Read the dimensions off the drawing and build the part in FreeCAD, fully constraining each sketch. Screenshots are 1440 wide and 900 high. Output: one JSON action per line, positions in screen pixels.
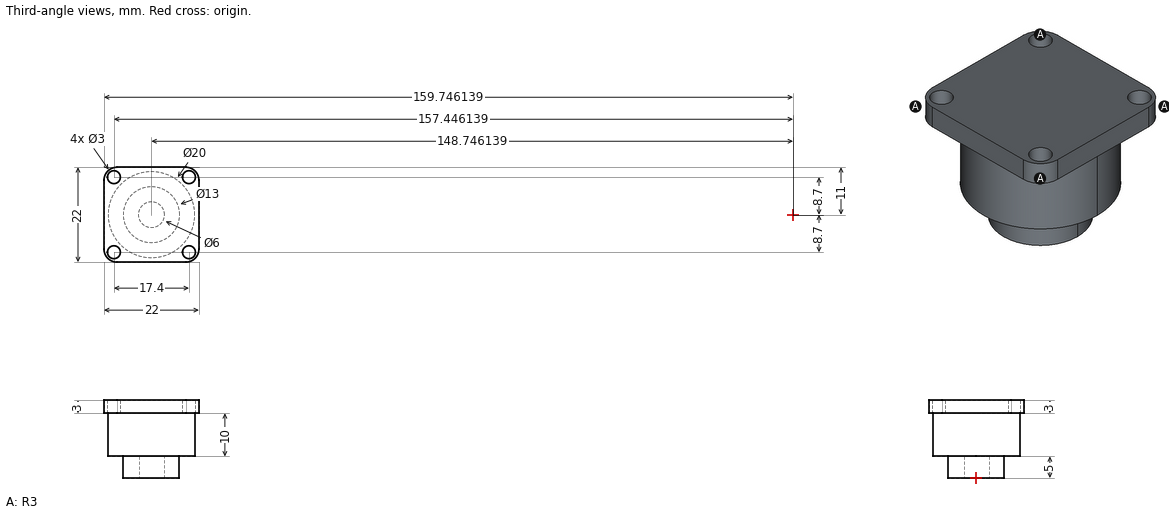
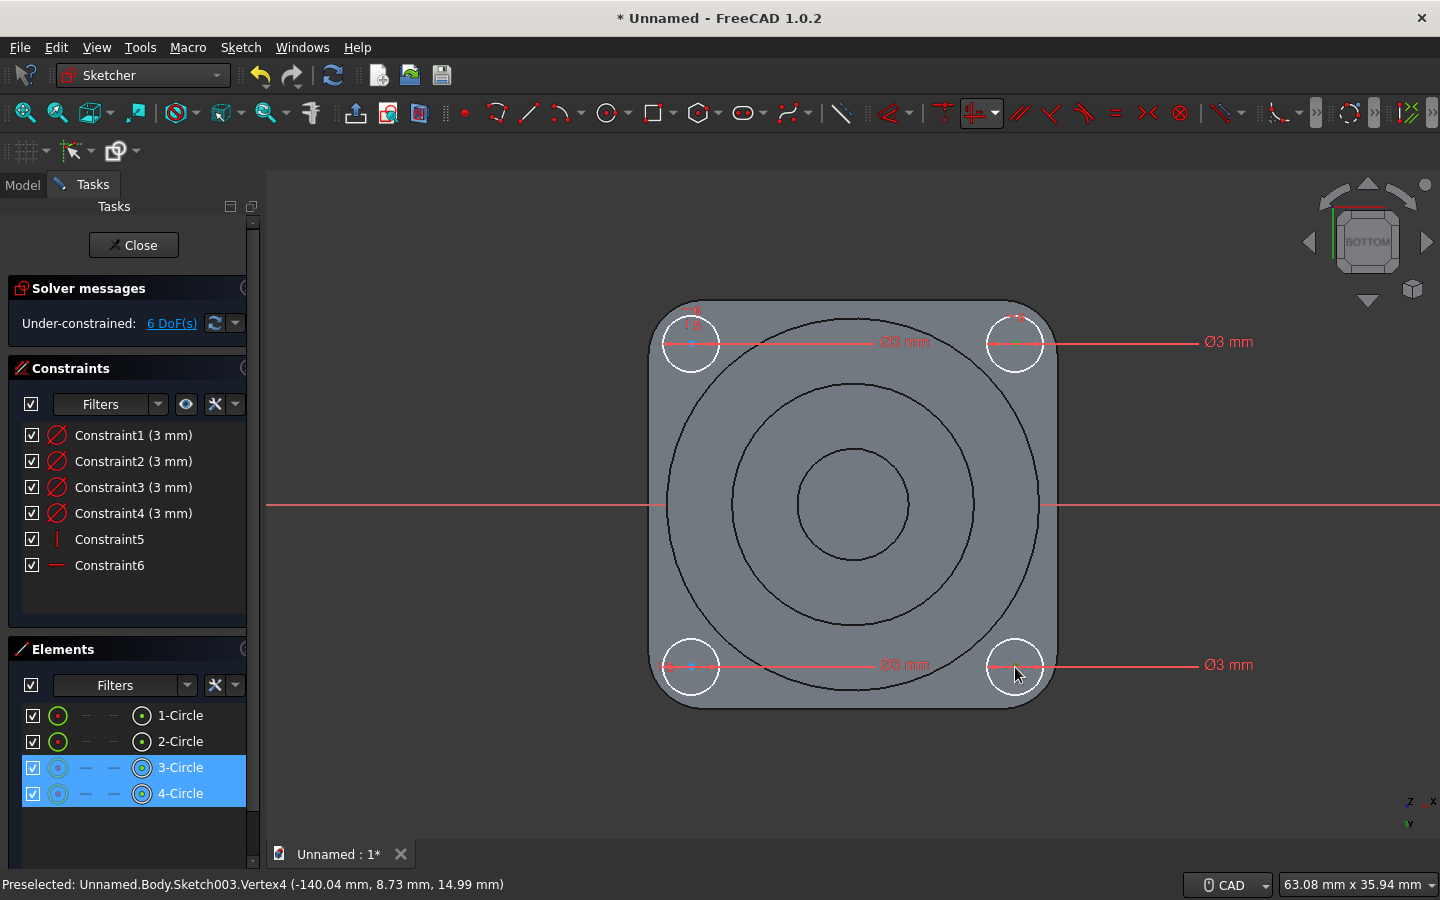
{"action": "left_click", "coordinate": [998, 114]}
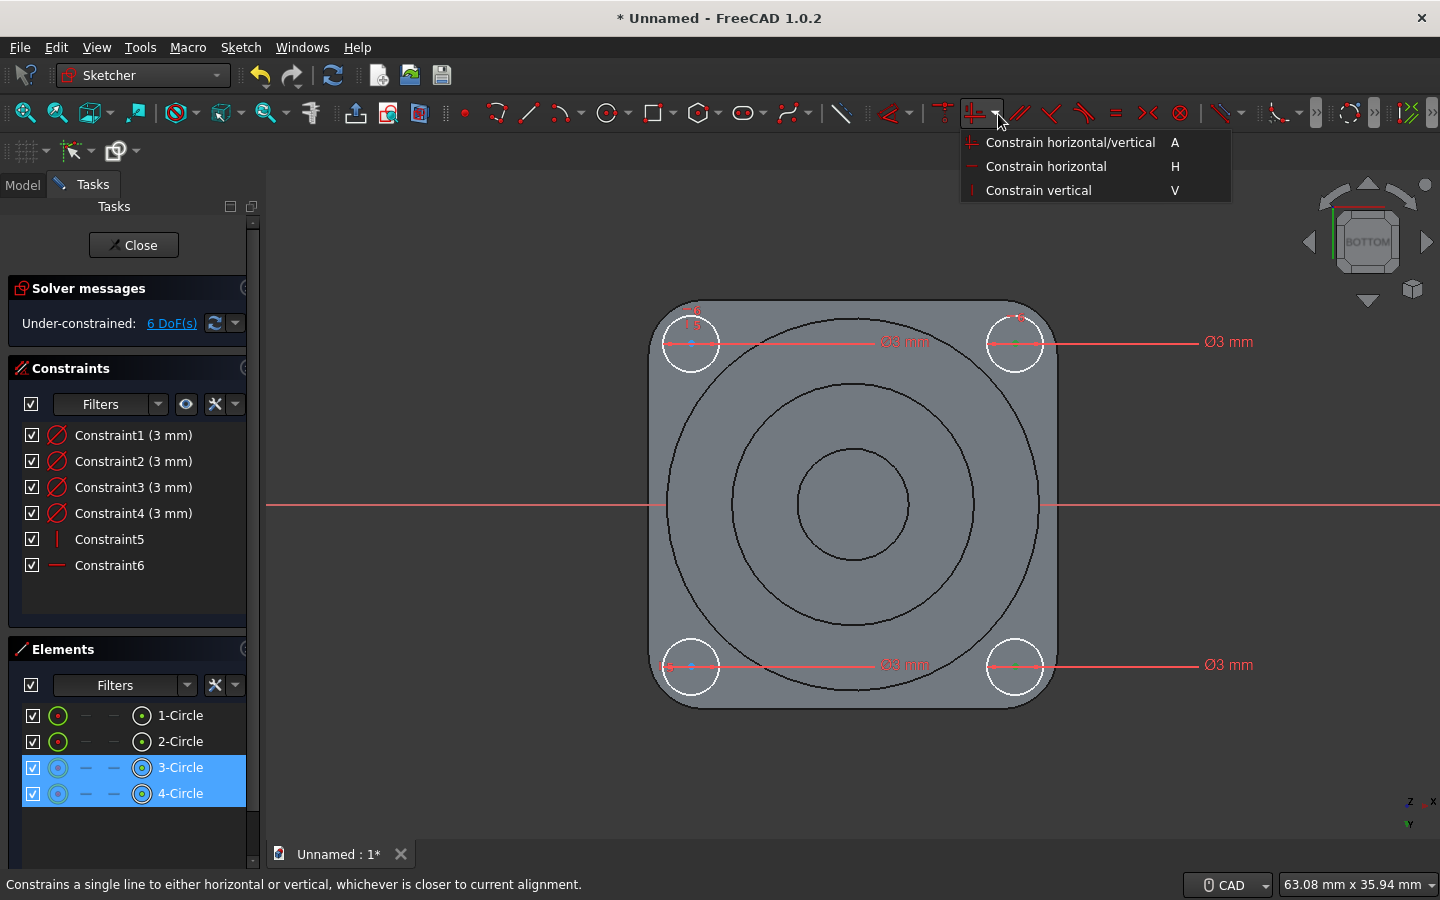
{"action": "left_click", "coordinate": [1096, 190]}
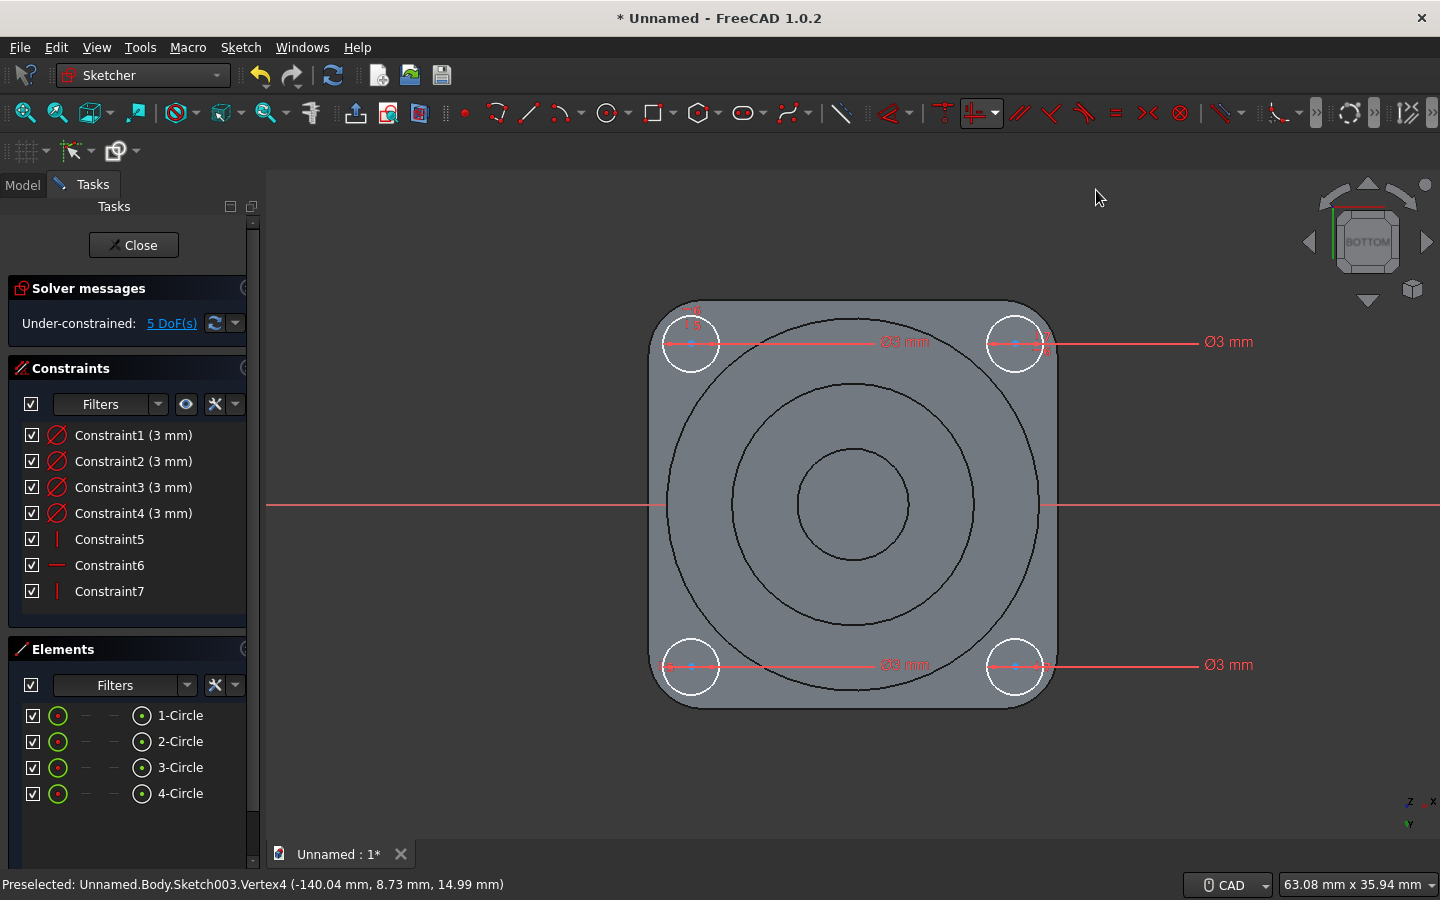
{"action": "left_click", "coordinate": [691, 667]}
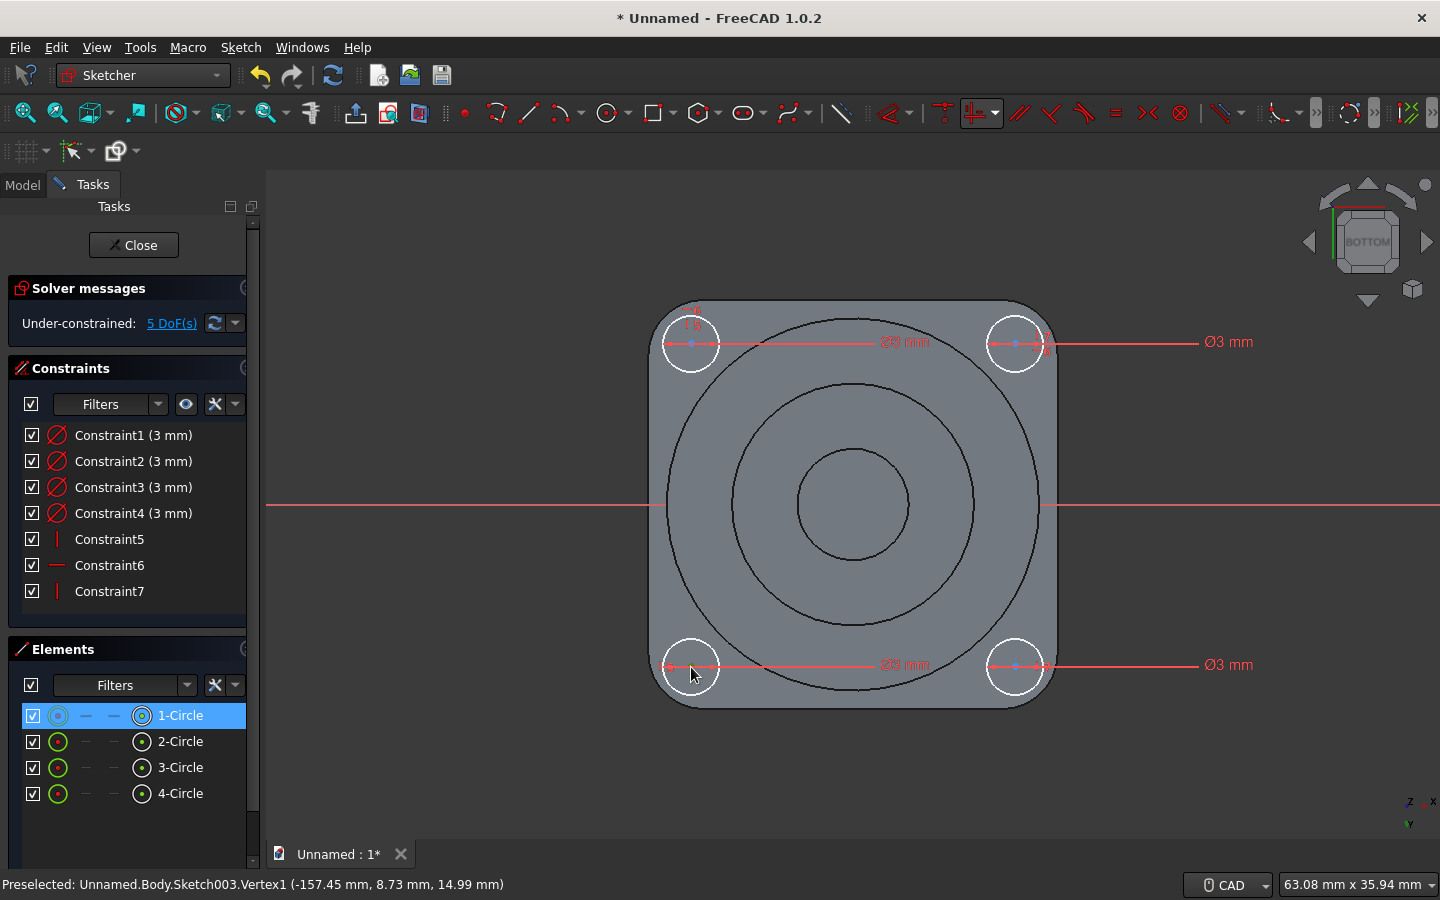
{"action": "left_click", "coordinate": [1015, 667]}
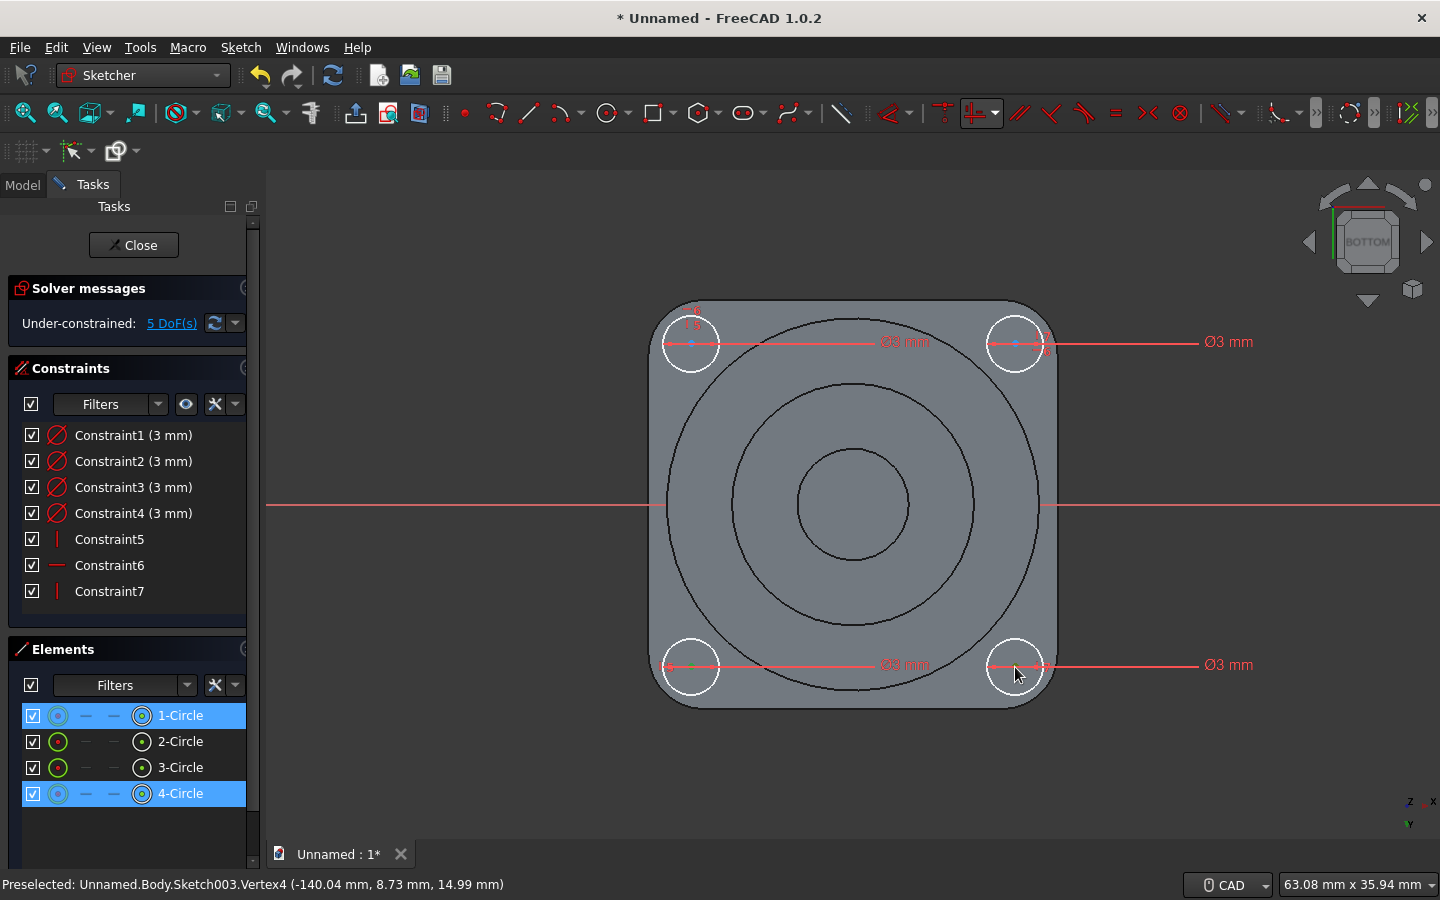
{"action": "left_click", "coordinate": [998, 114]}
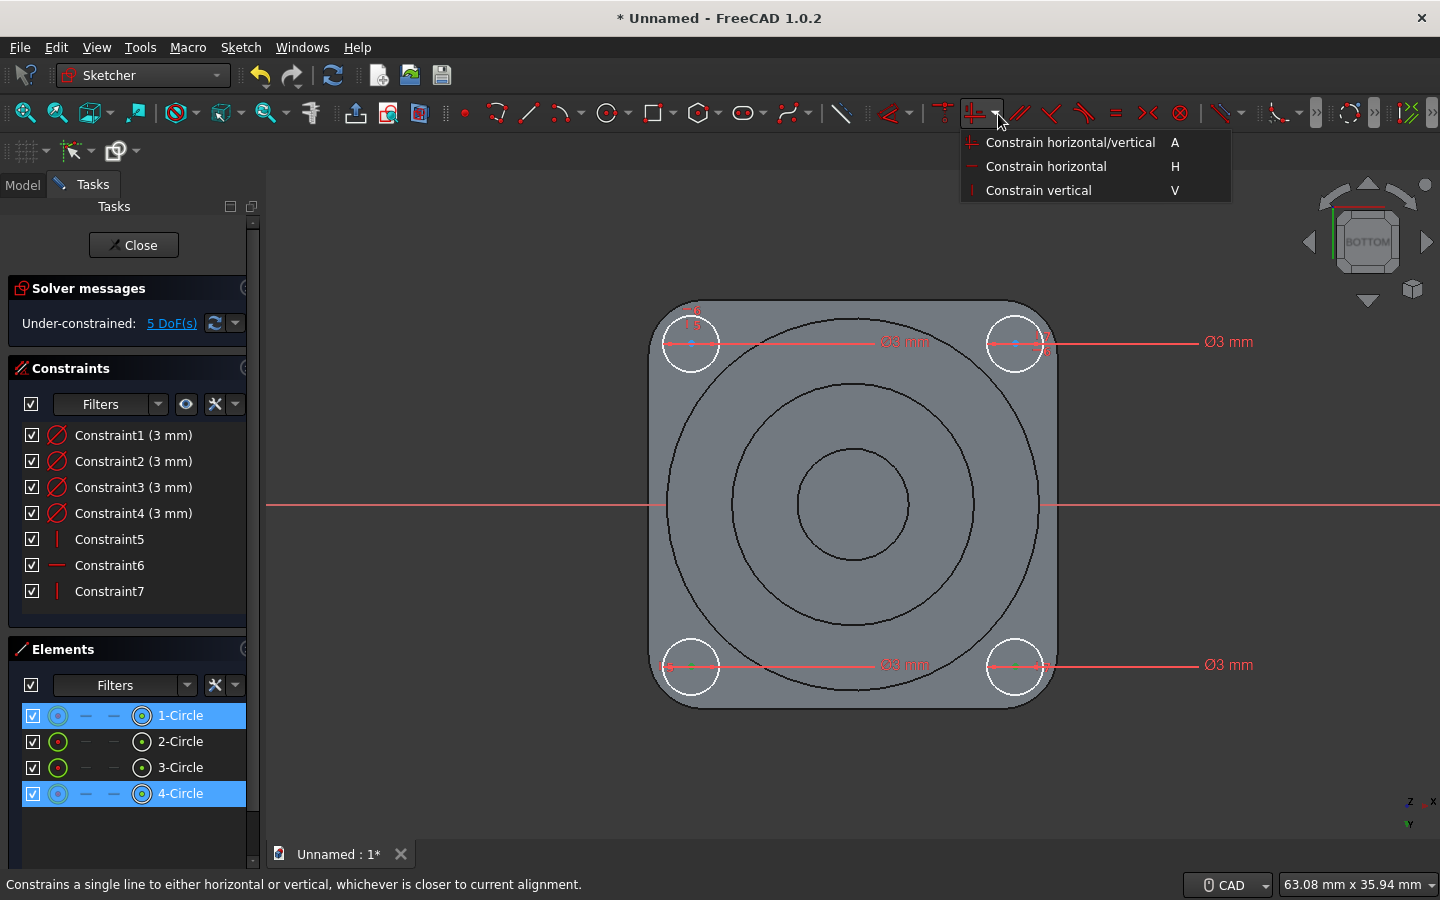
{"action": "left_click", "coordinate": [1096, 166]}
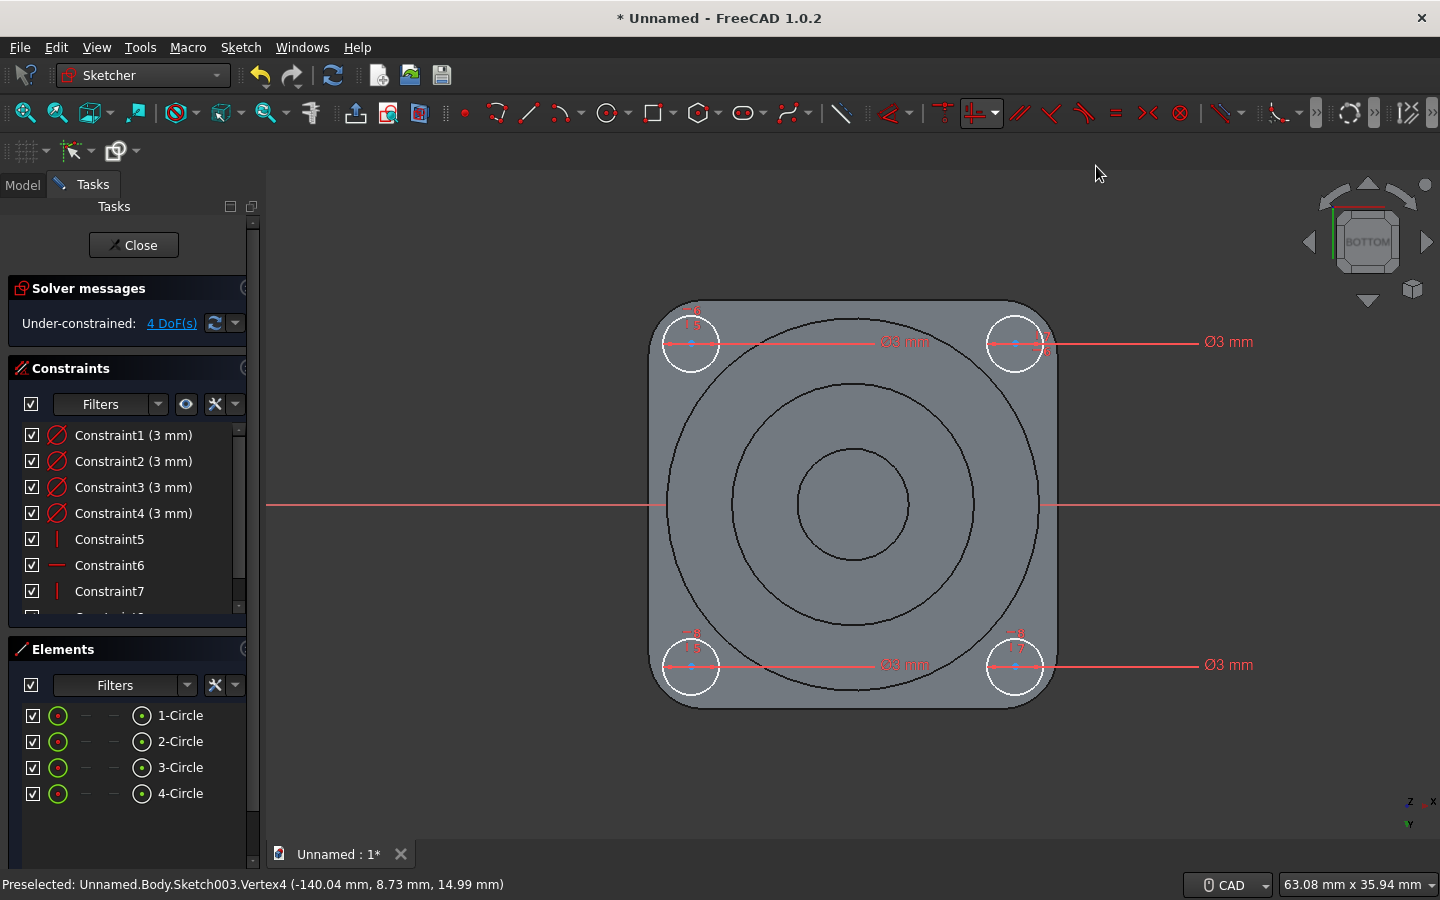
{"action": "key", "text": "d"}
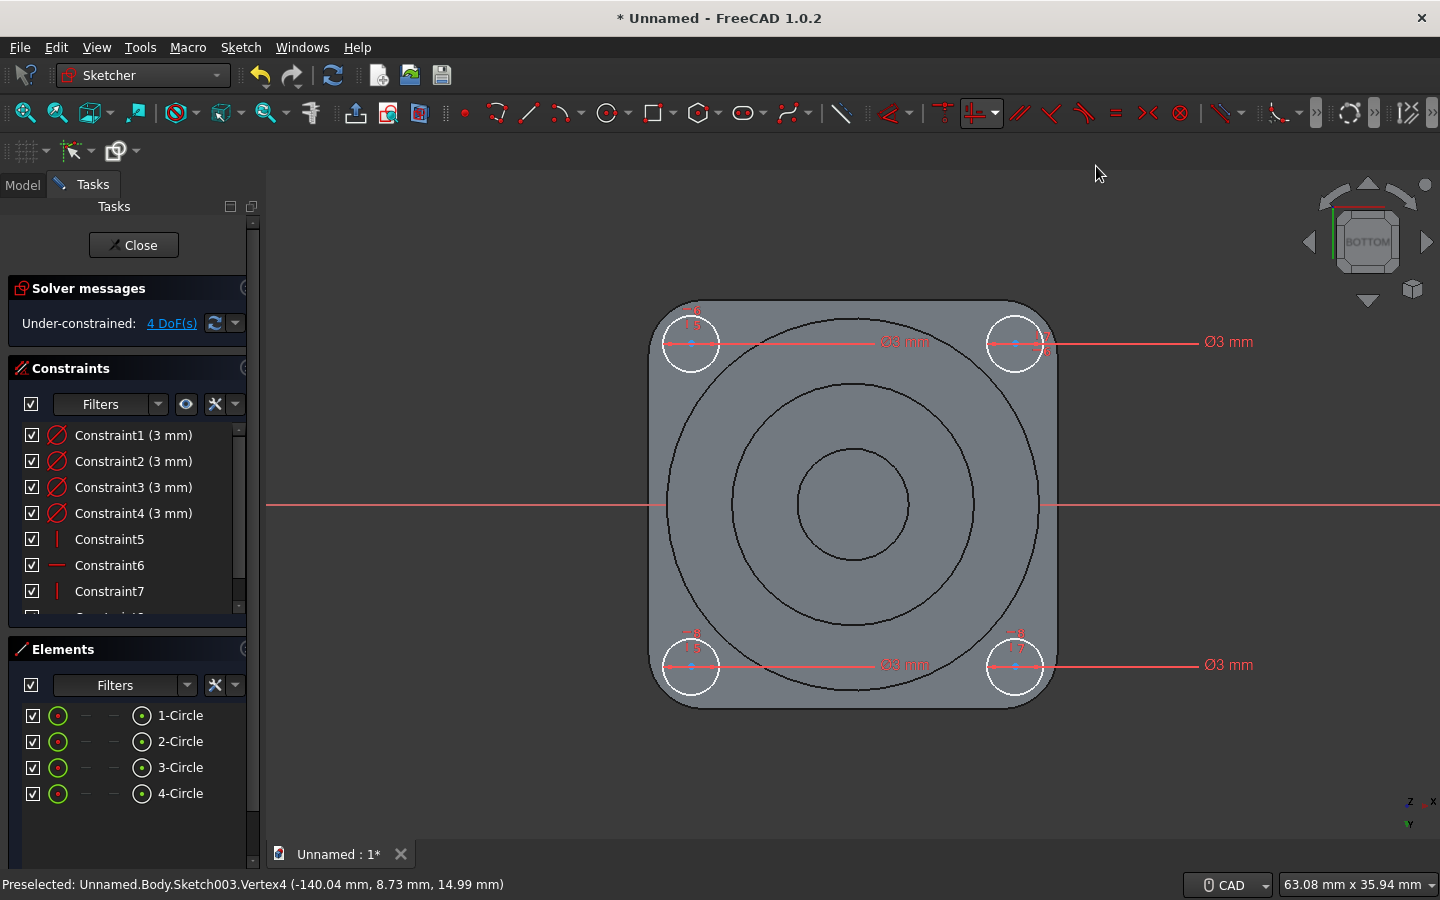
{"action": "left_click", "coordinate": [691, 667]}
{"action": "left_click", "coordinate": [657, 586]}